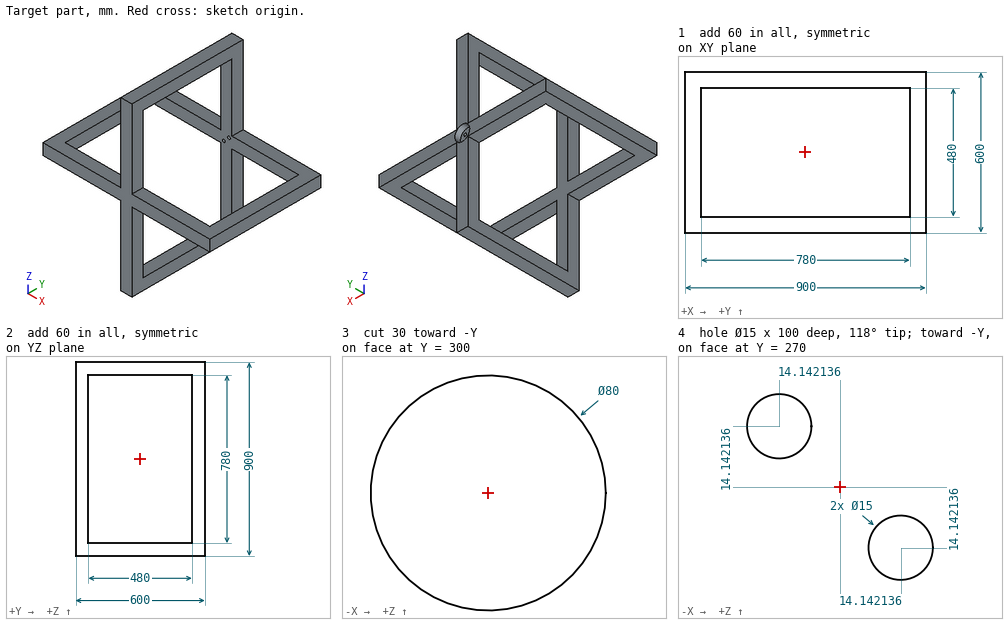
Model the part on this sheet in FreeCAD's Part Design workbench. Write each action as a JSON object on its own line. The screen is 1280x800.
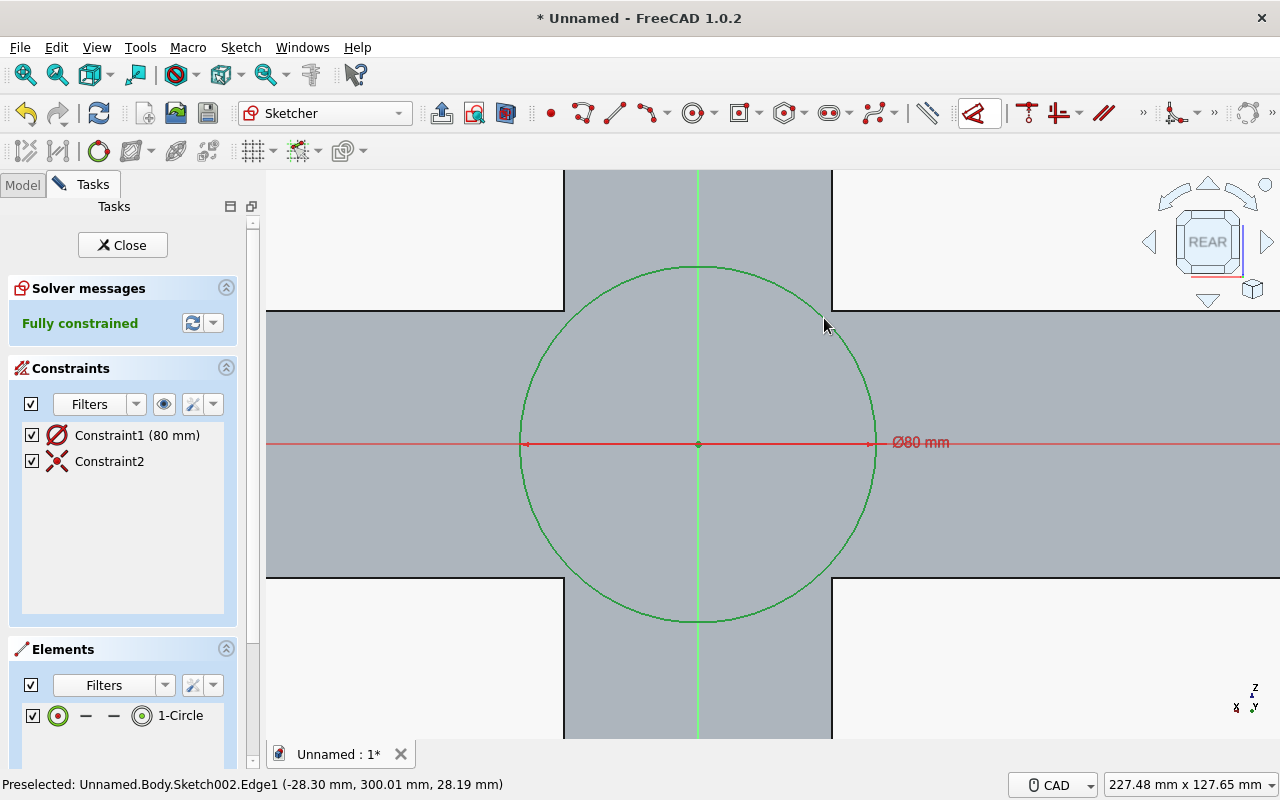
{"action": "left_click", "coordinate": [123, 245]}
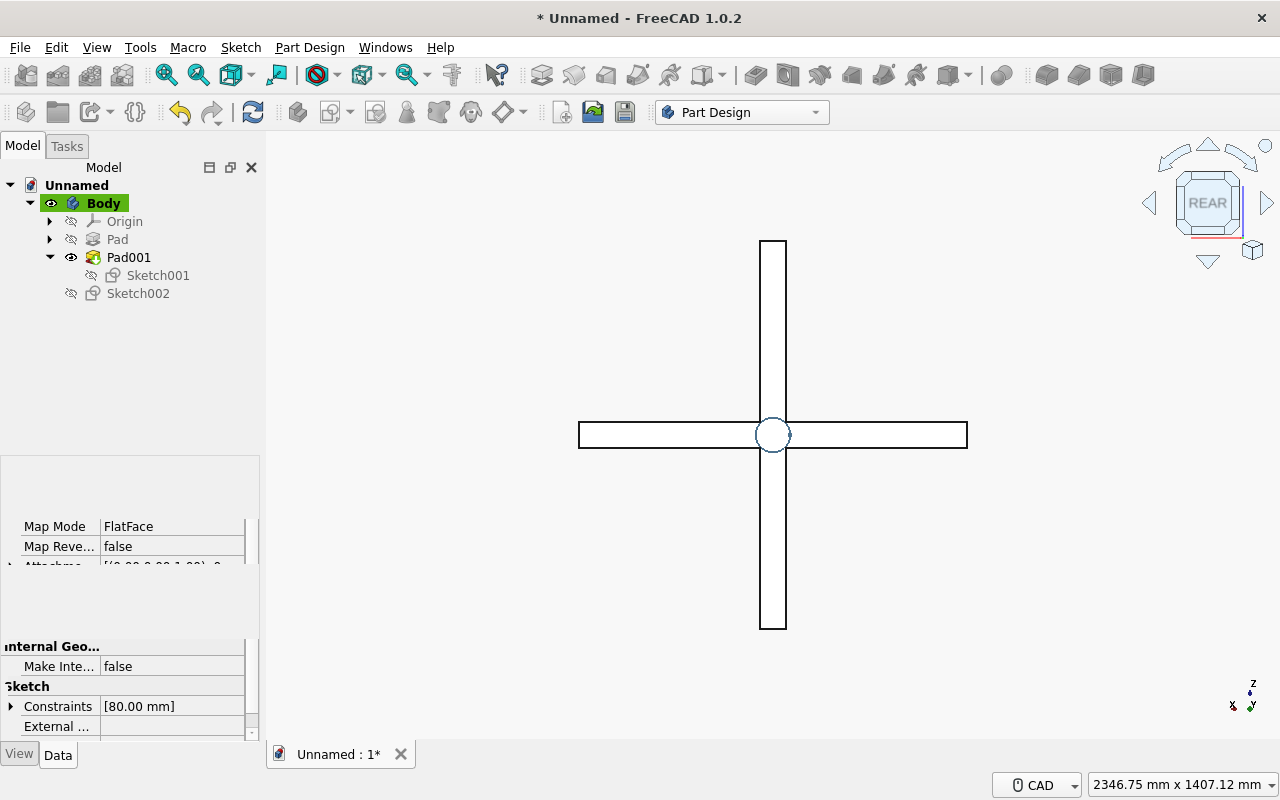
{"action": "left_click", "coordinate": [756, 76]}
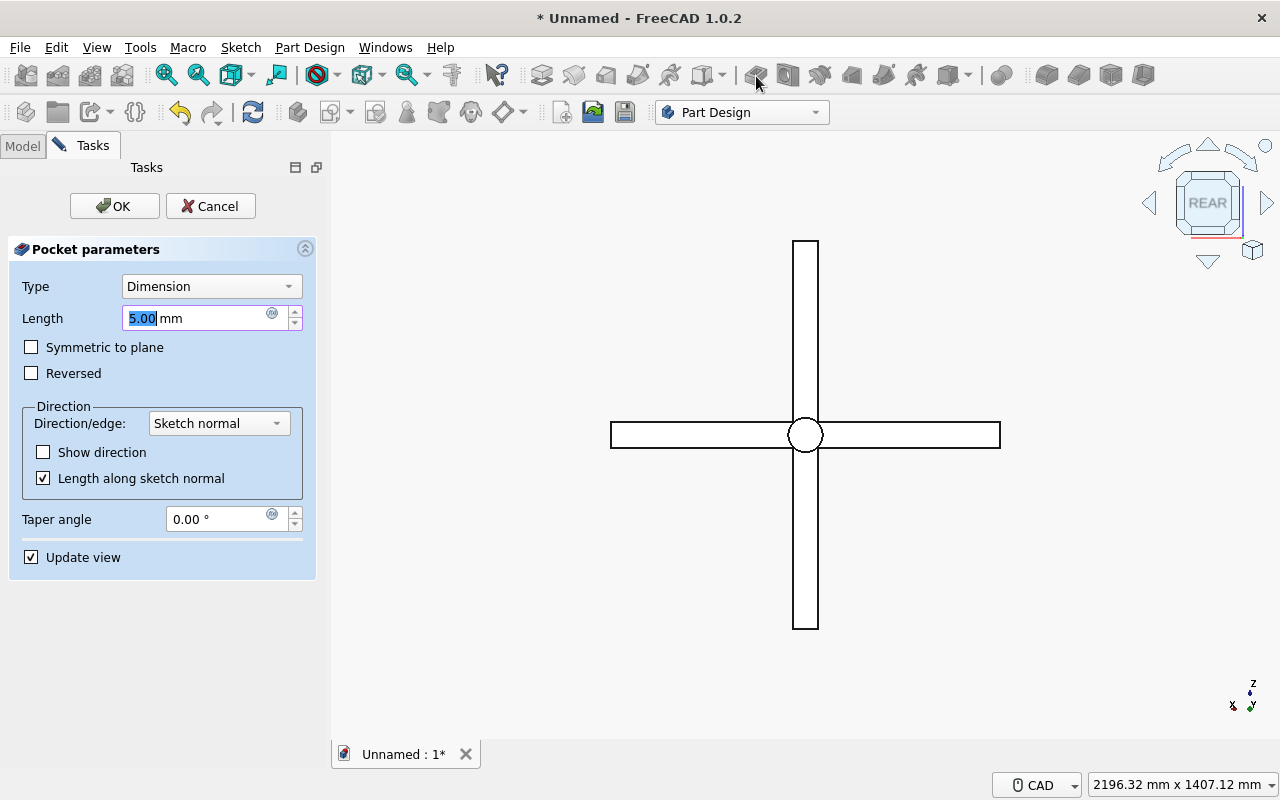
{"action": "type", "text": "30"}
{"action": "key", "text": "Tab"}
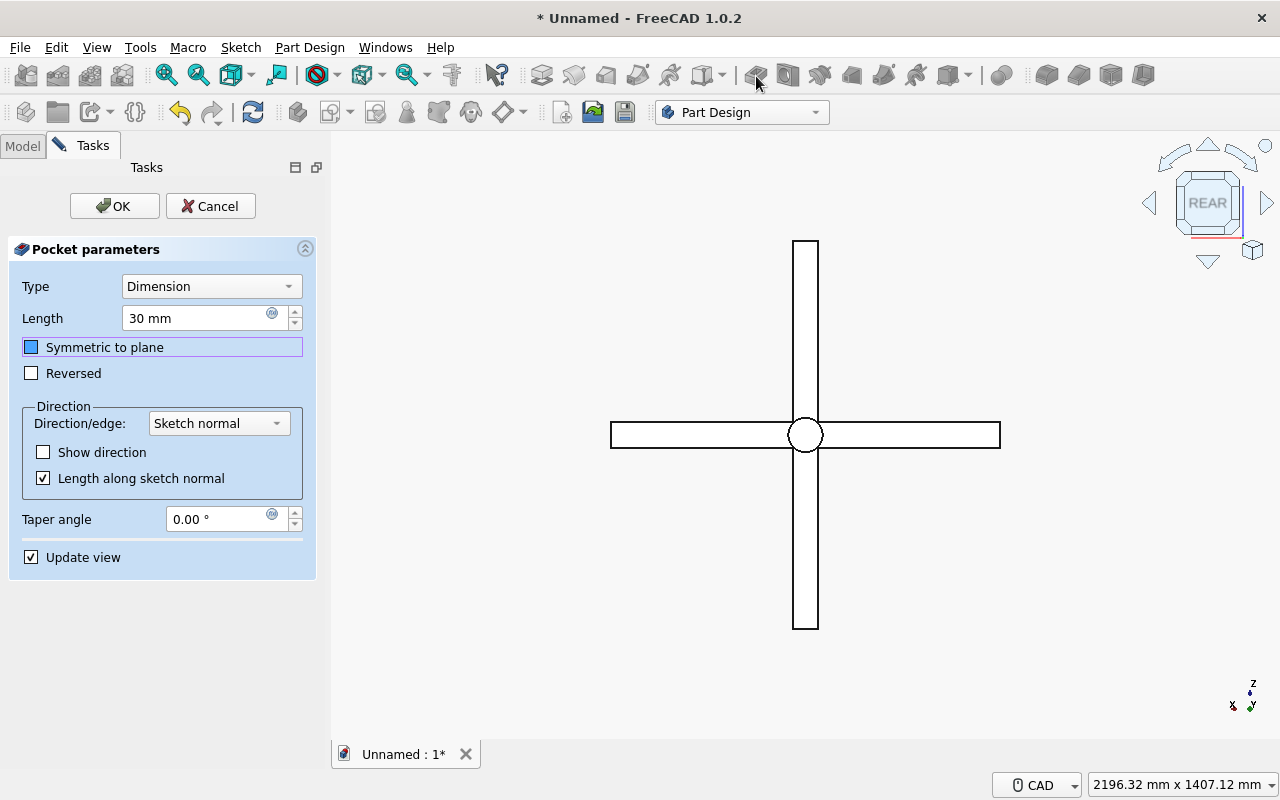
{"action": "left_click", "coordinate": [115, 206]}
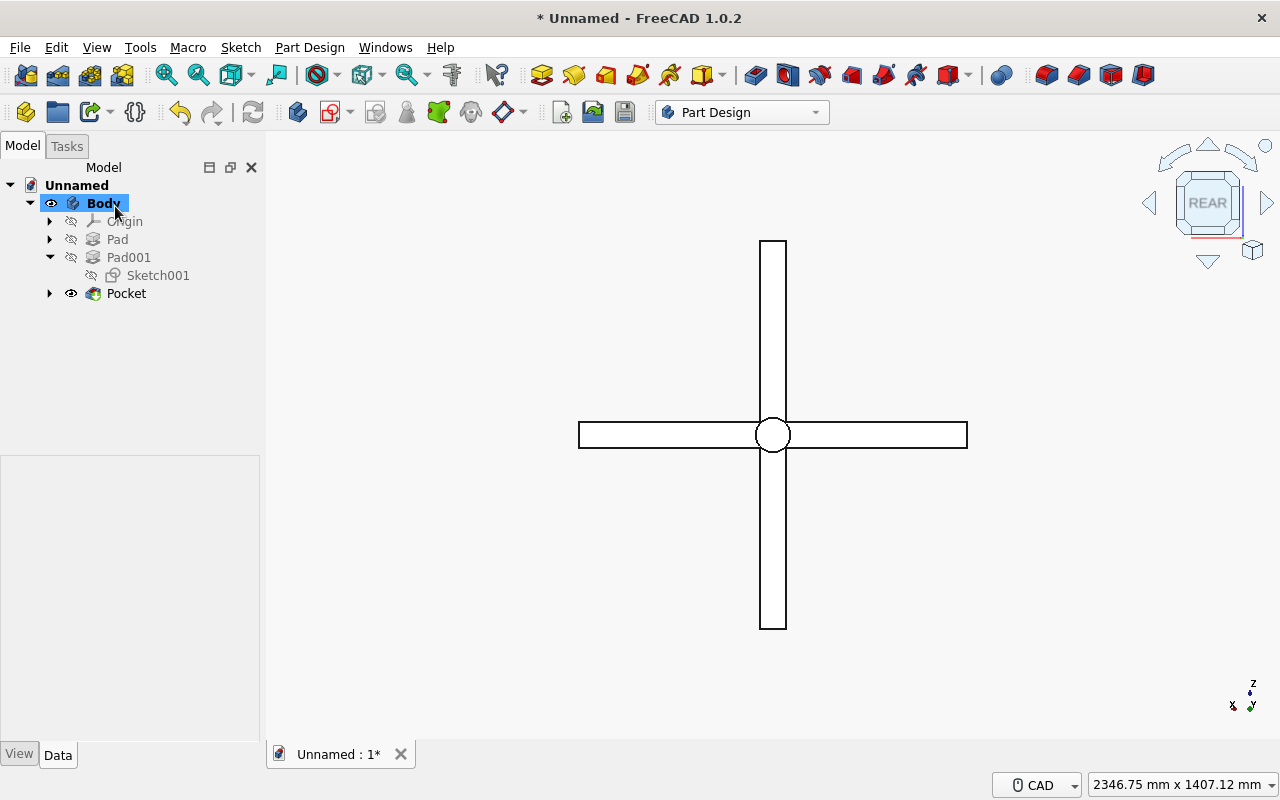
{"action": "left_click", "coordinate": [773, 434]}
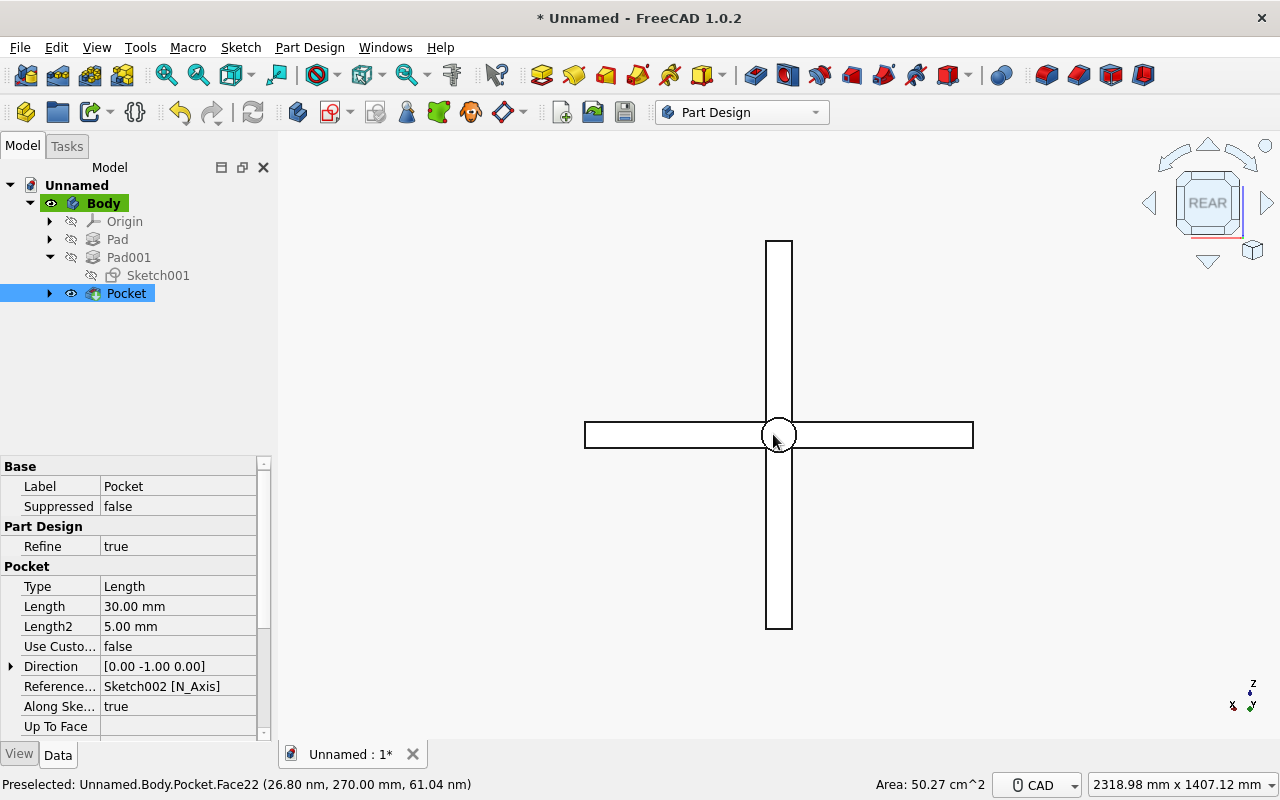
{"action": "left_click", "coordinate": [330, 112]}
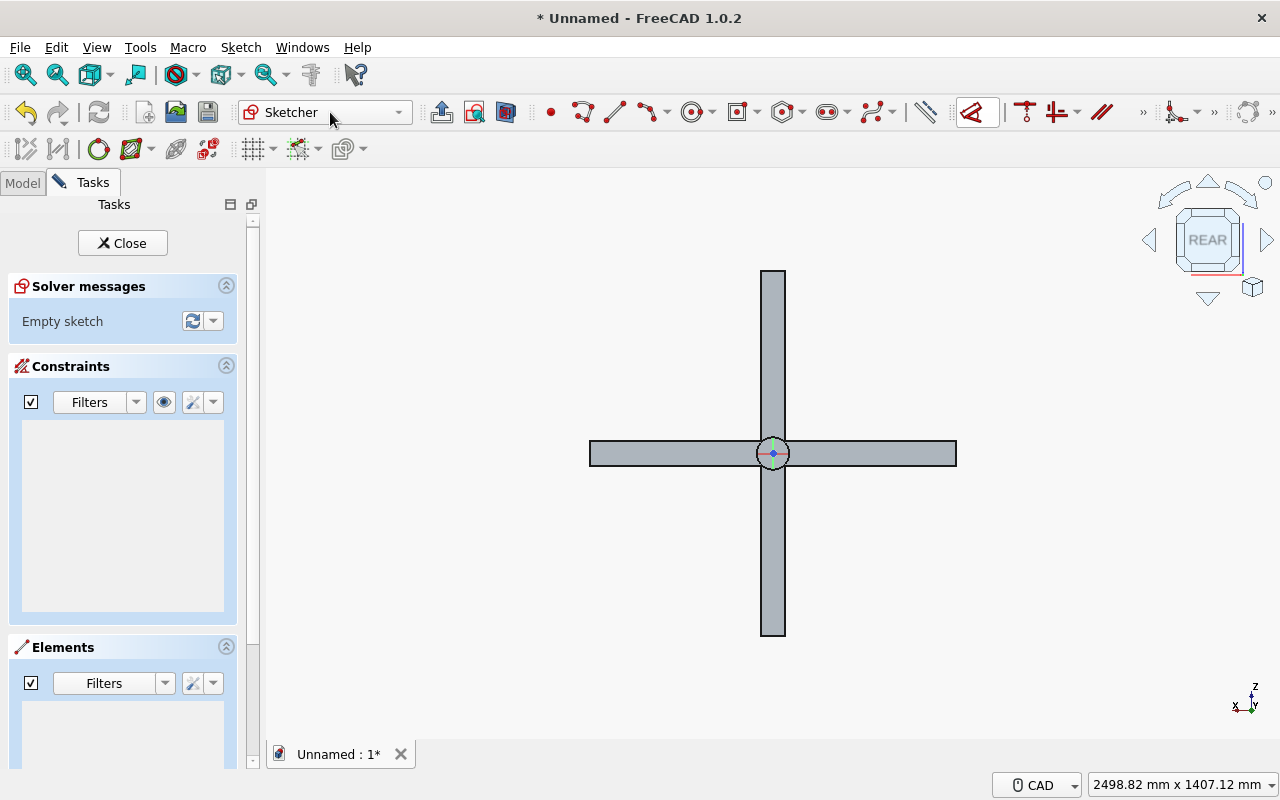
{"action": "scroll", "coordinate": [777, 454], "scroll_direction": "up", "scroll_amount": 15}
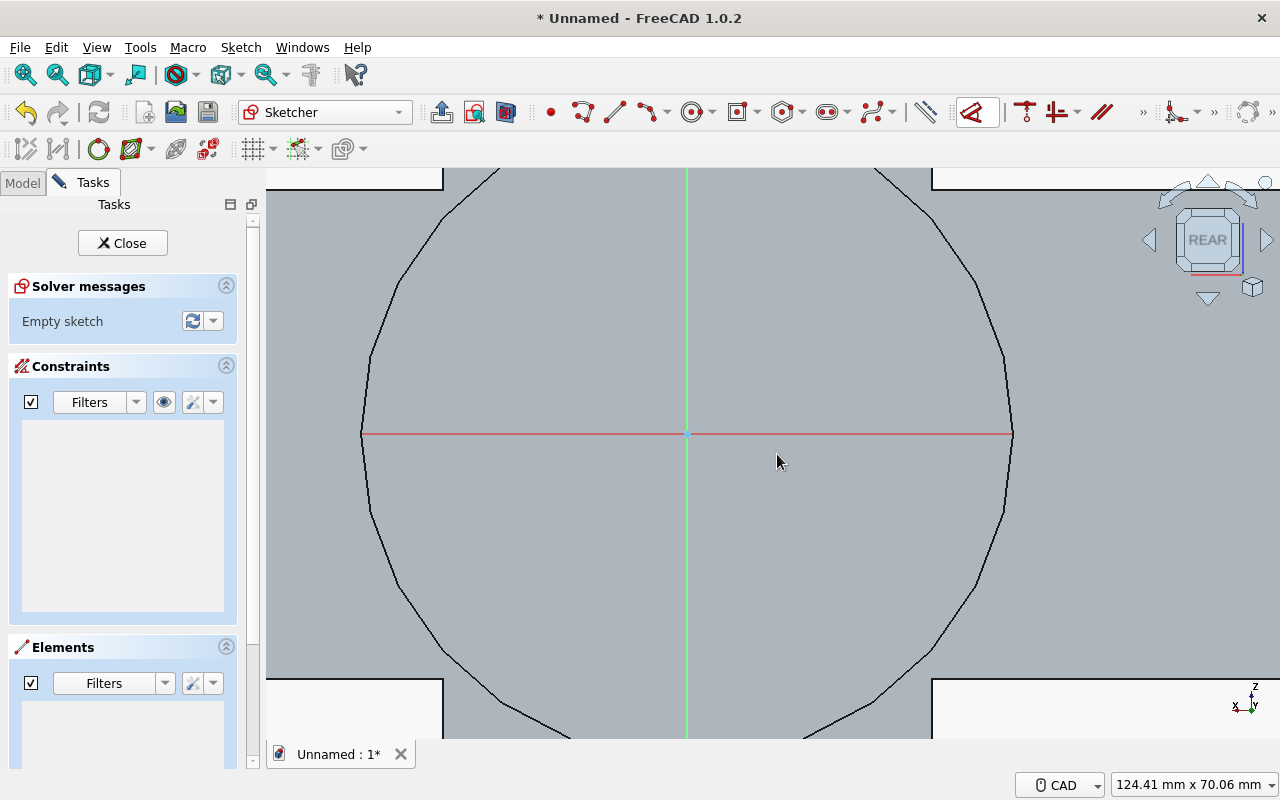
{"action": "left_click", "coordinate": [692, 112]}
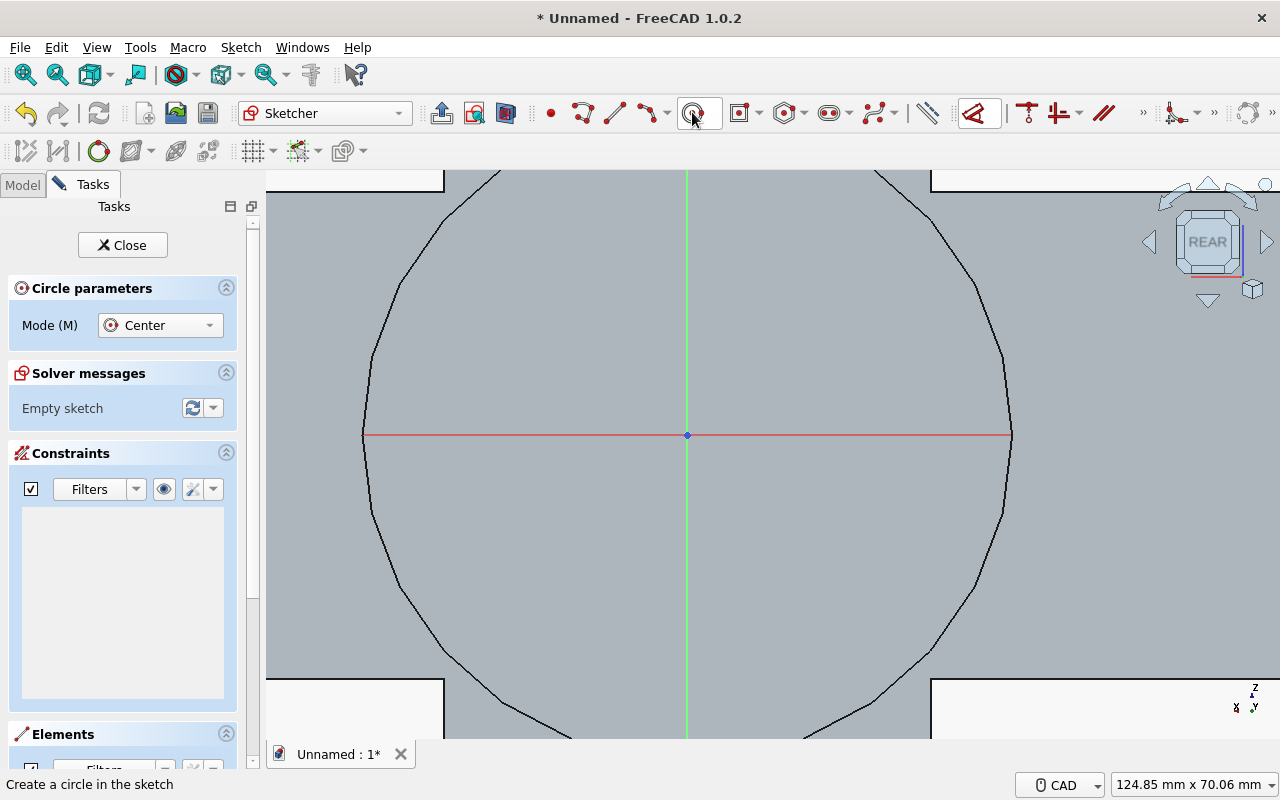
{"action": "left_click", "coordinate": [802, 550]}
{"action": "mouse_move", "coordinate": [845, 507]}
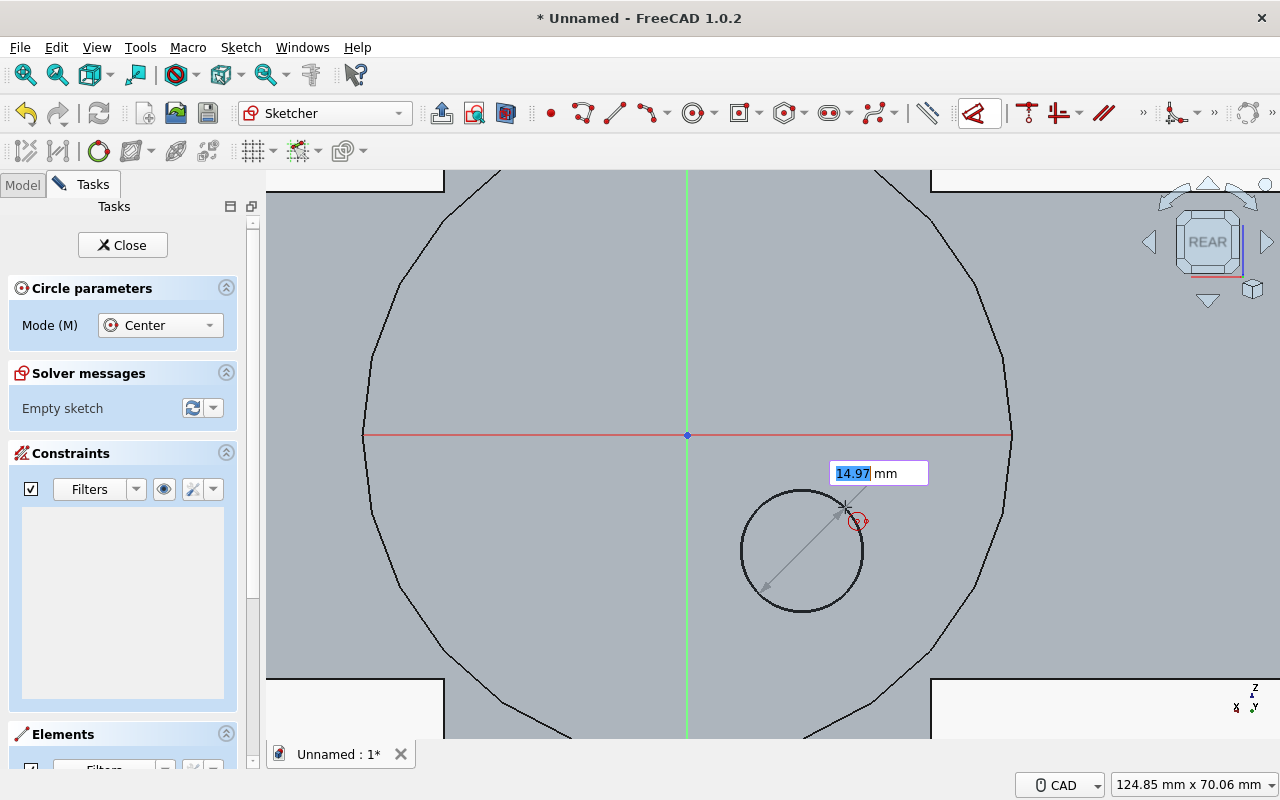
{"action": "type", "text": "15"}
{"action": "key", "text": "Return"}